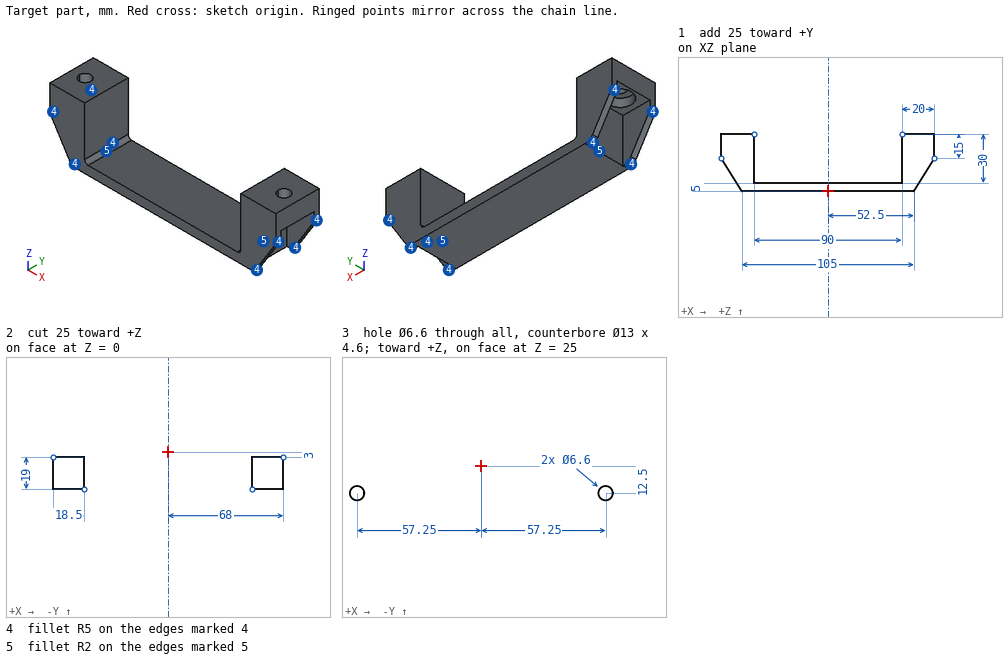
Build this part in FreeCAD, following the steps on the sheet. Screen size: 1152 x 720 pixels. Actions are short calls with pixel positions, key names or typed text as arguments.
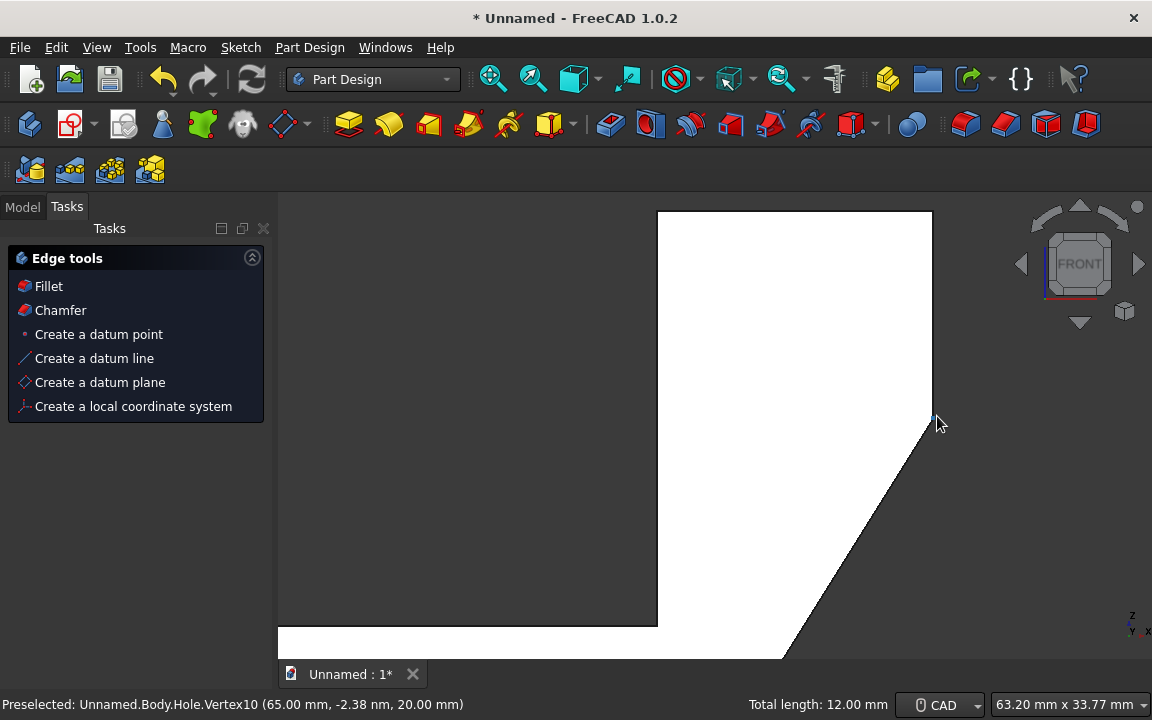
click(494, 80)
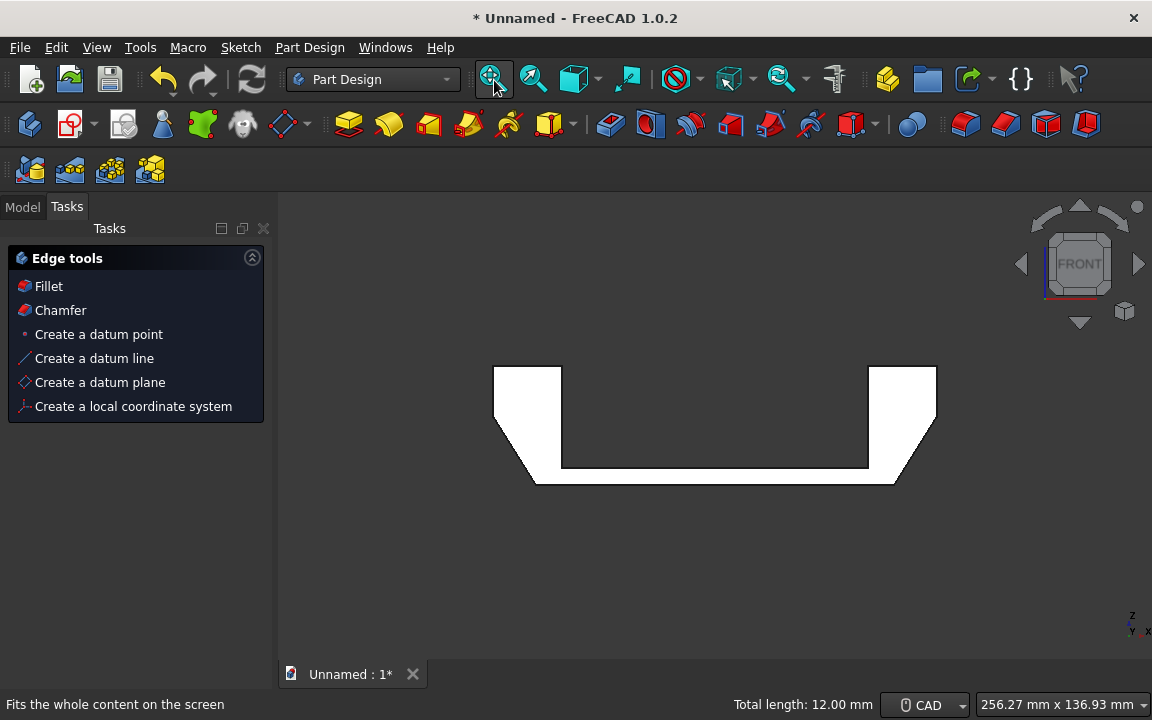
key(3)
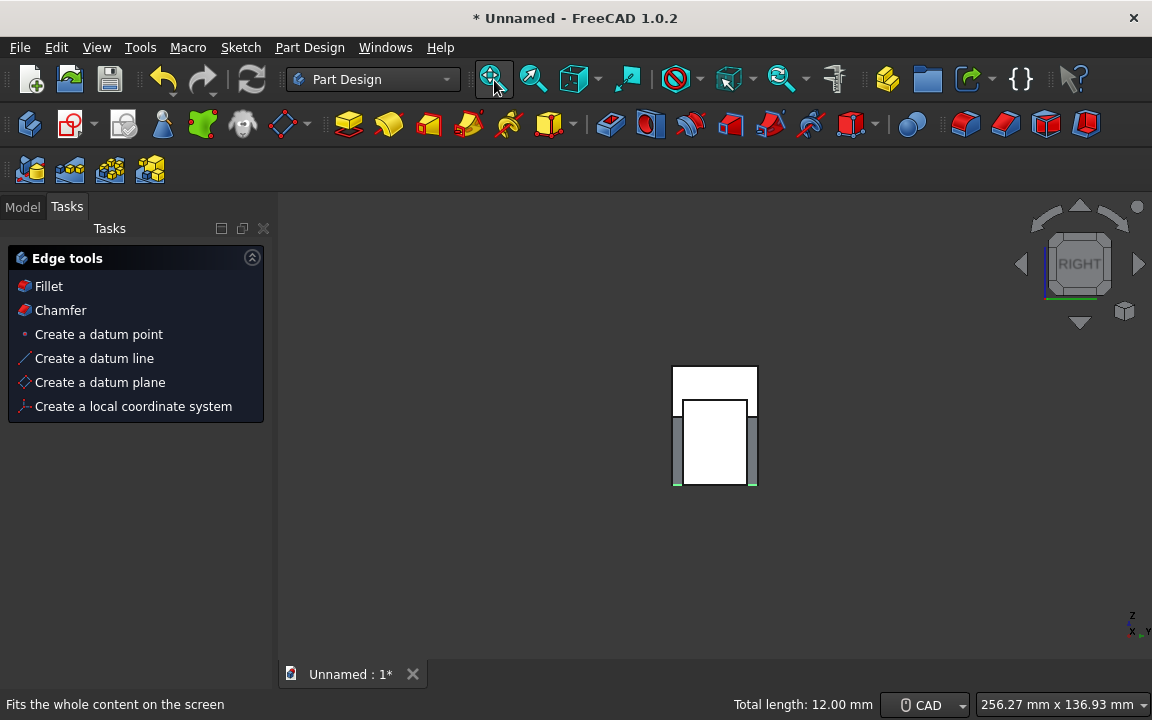
click(494, 80)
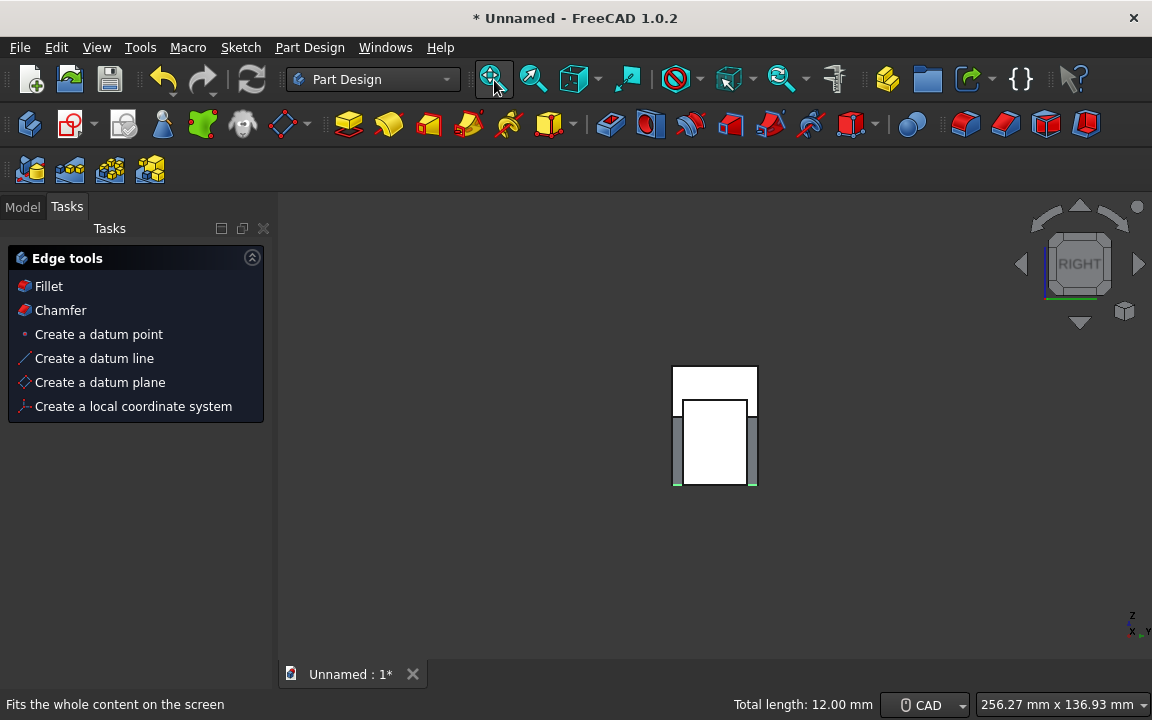
scroll(753, 416, up, 7)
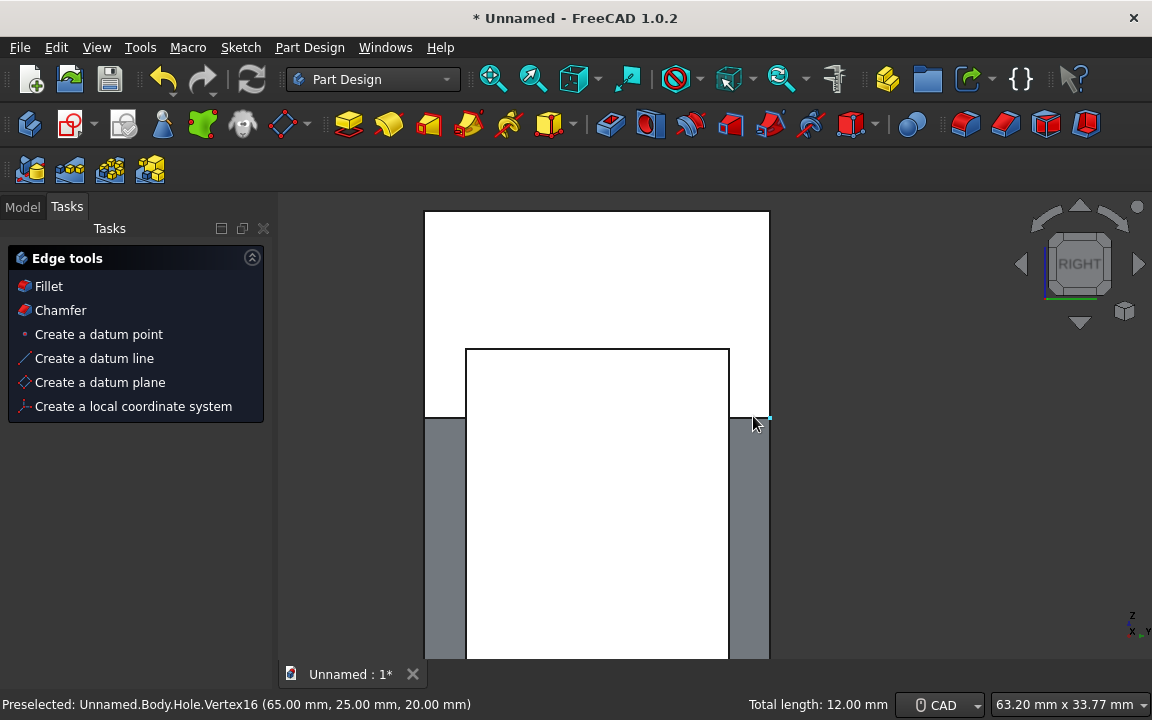
click(749, 417, ctrl)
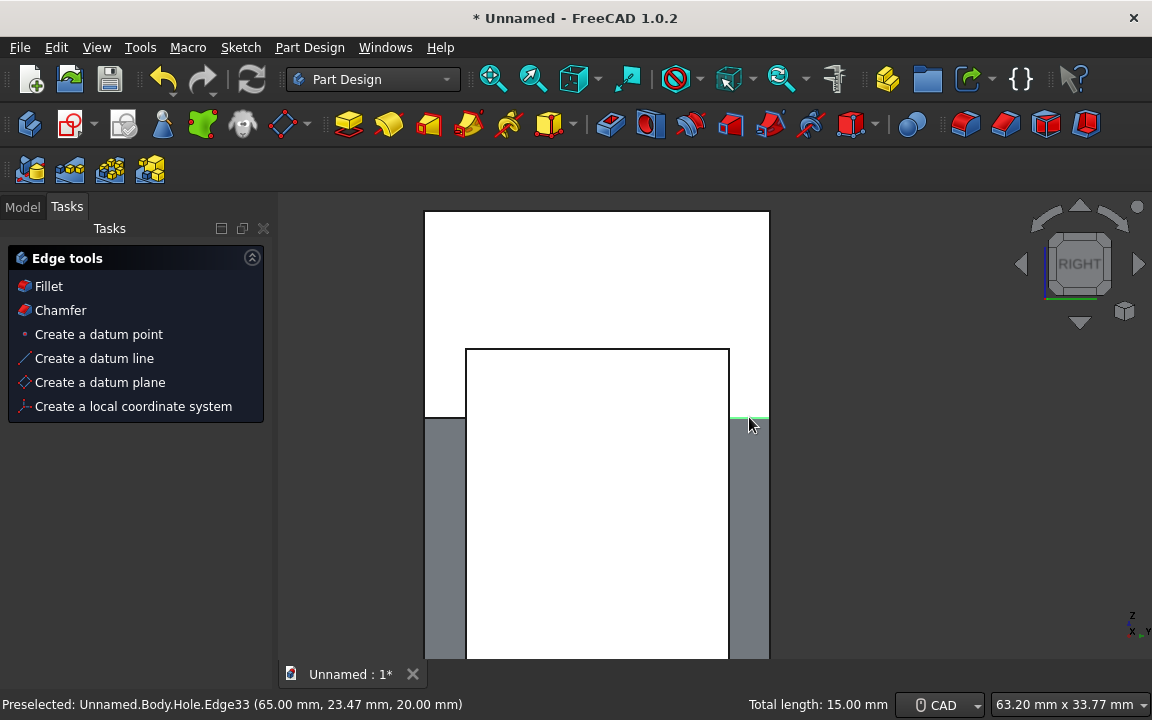
click(445, 417, ctrl)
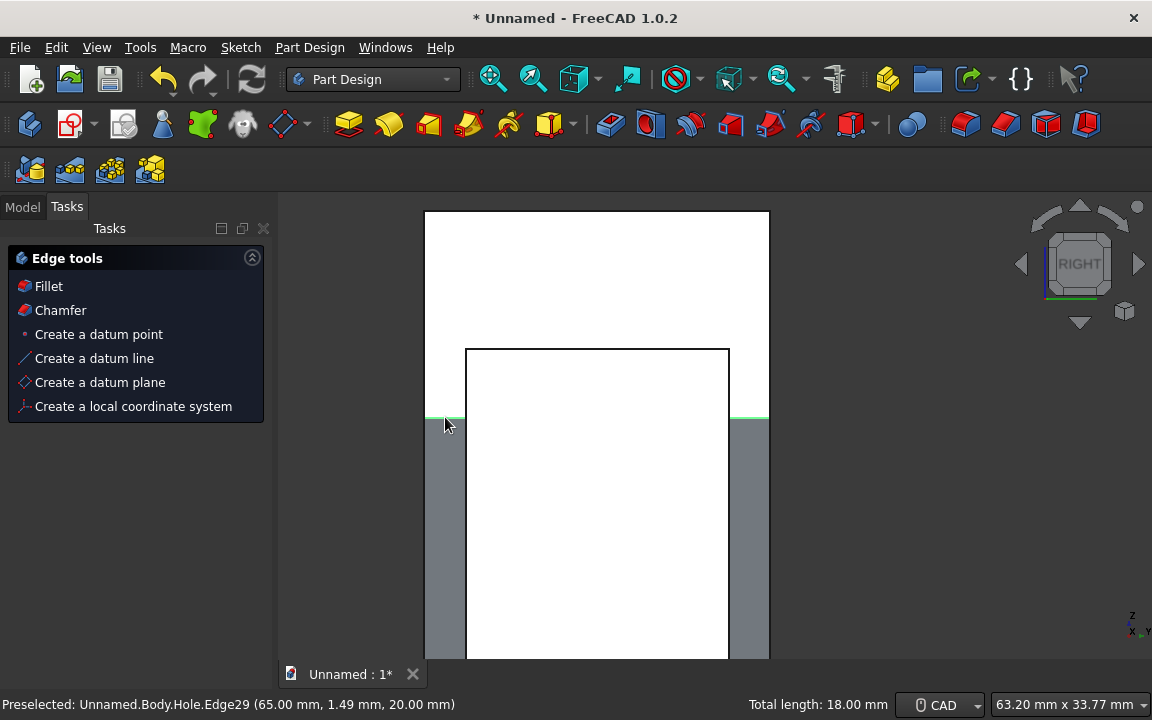
click(494, 80)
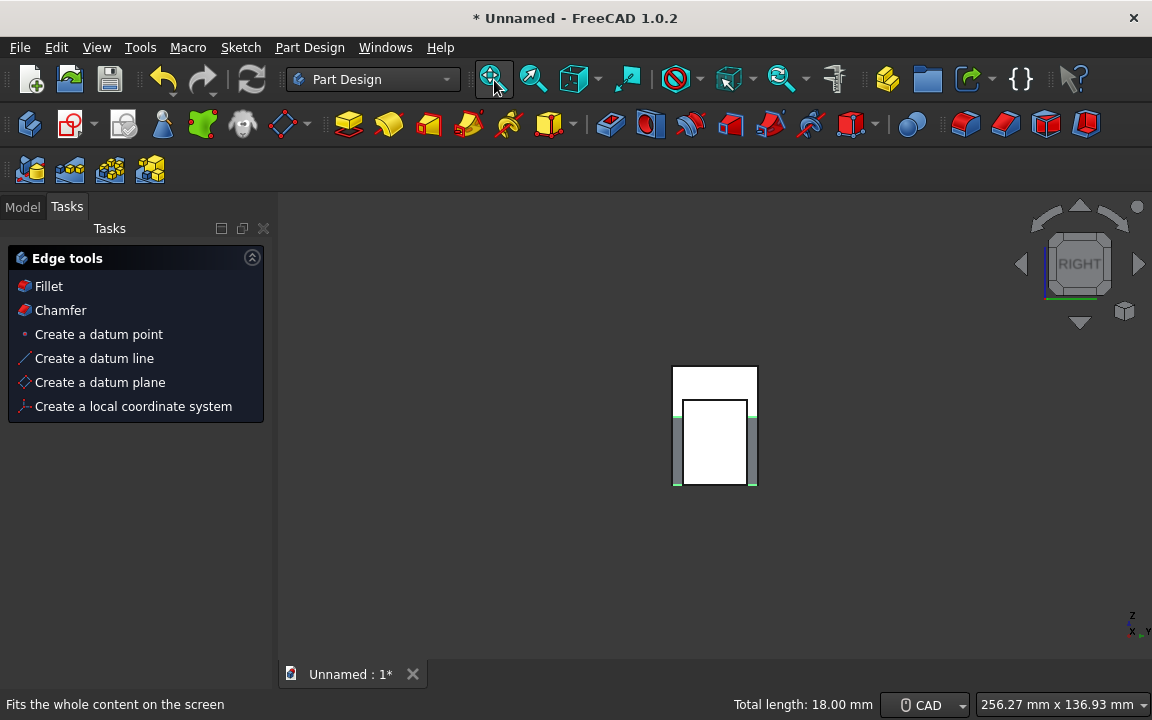
key(5)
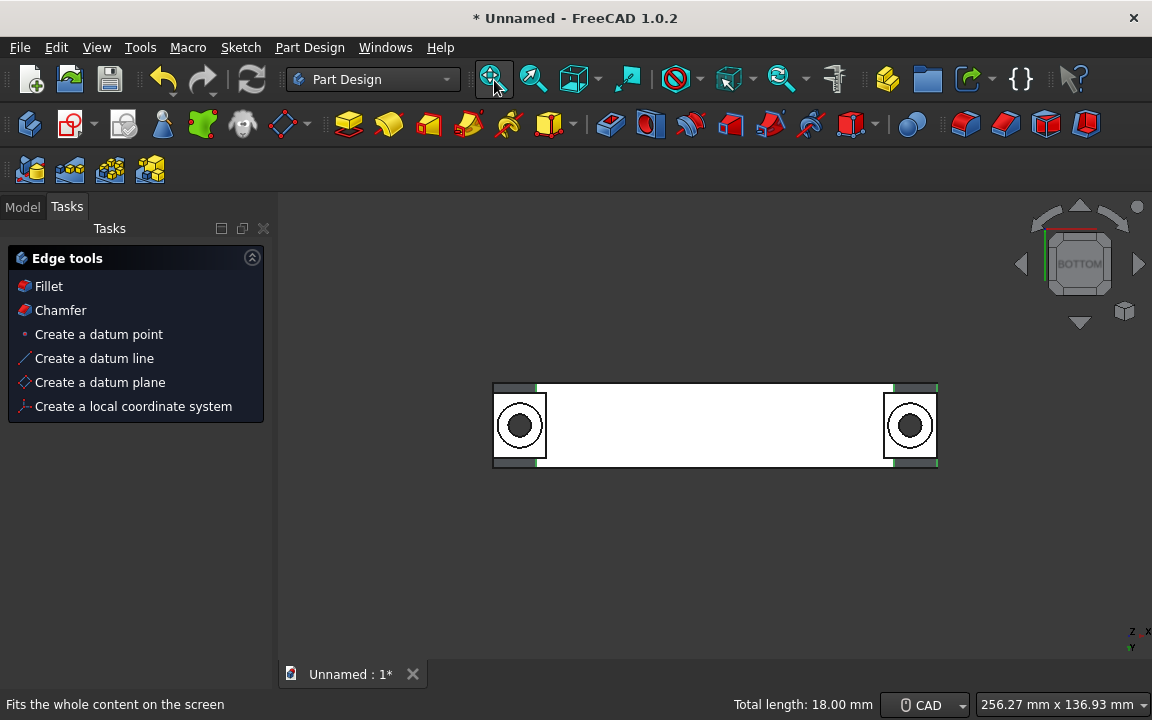
scroll(493, 462, up, 7)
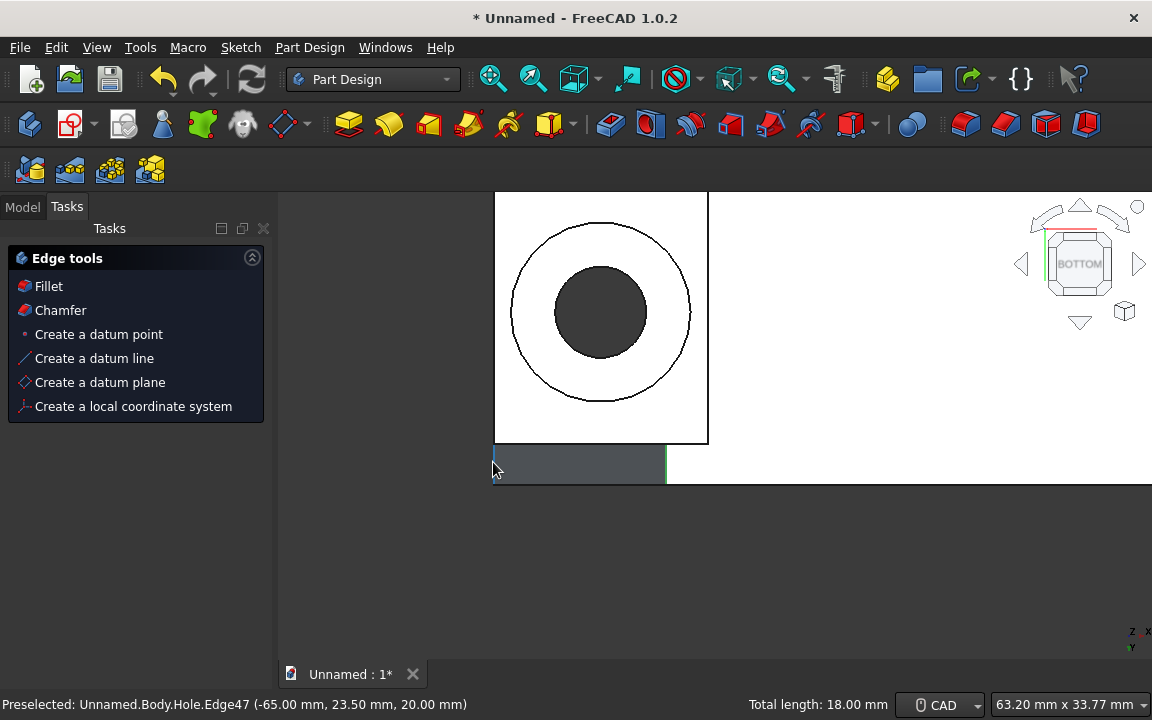
click(494, 80)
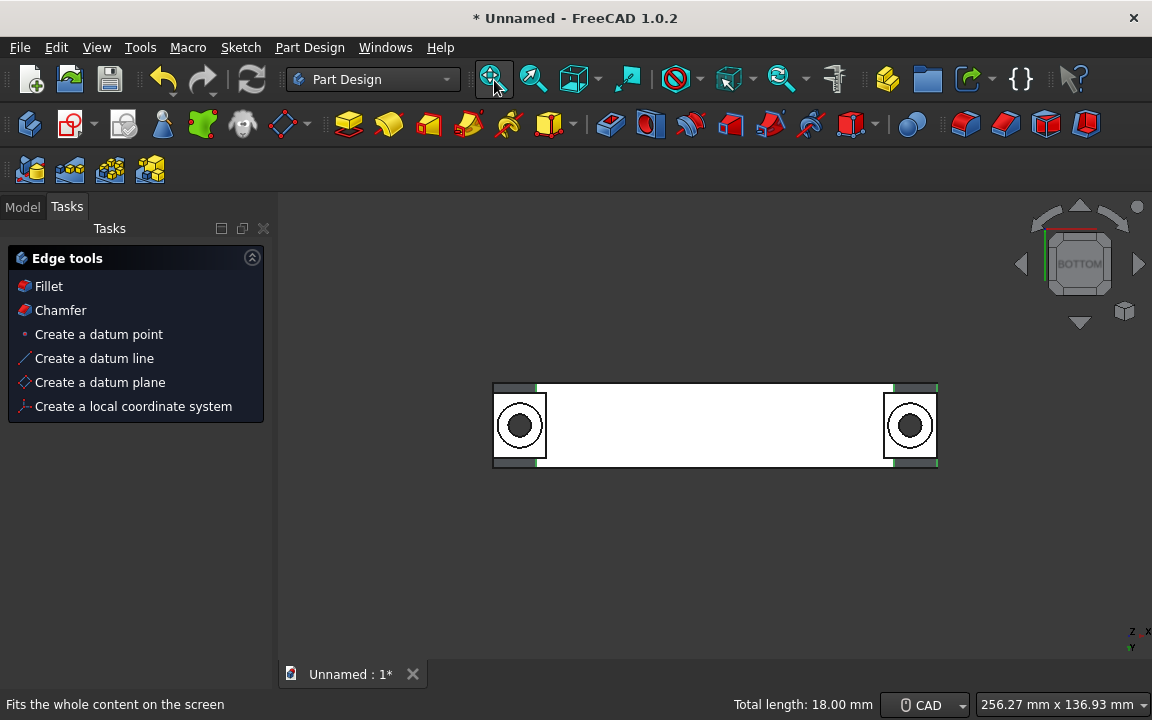
key(4)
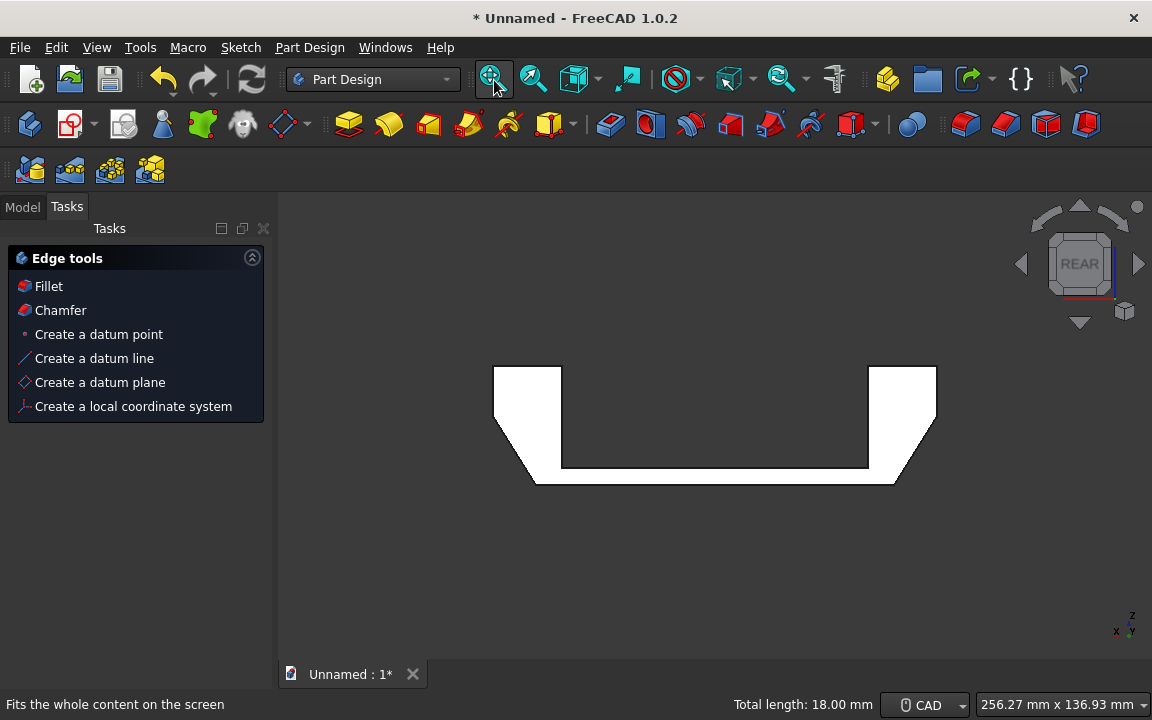
scroll(937, 416, up, 7)